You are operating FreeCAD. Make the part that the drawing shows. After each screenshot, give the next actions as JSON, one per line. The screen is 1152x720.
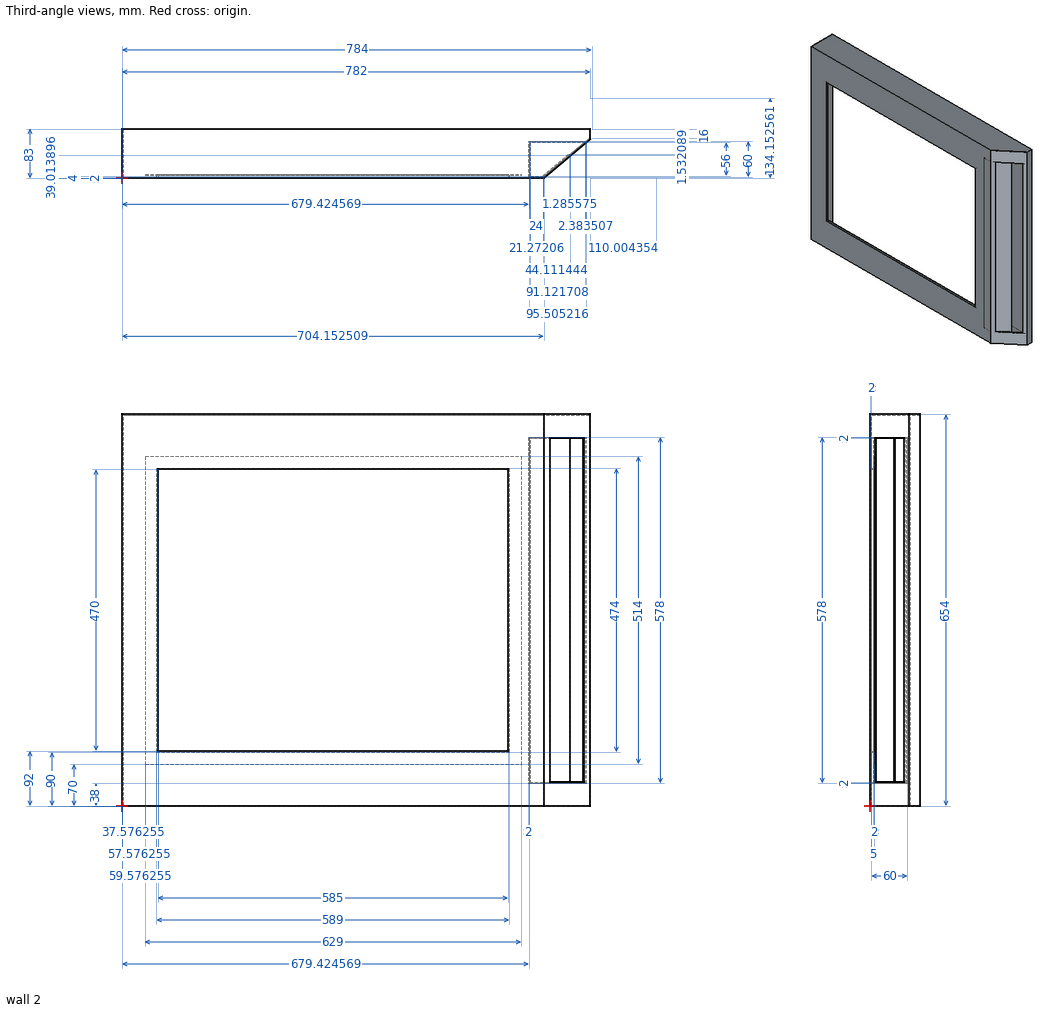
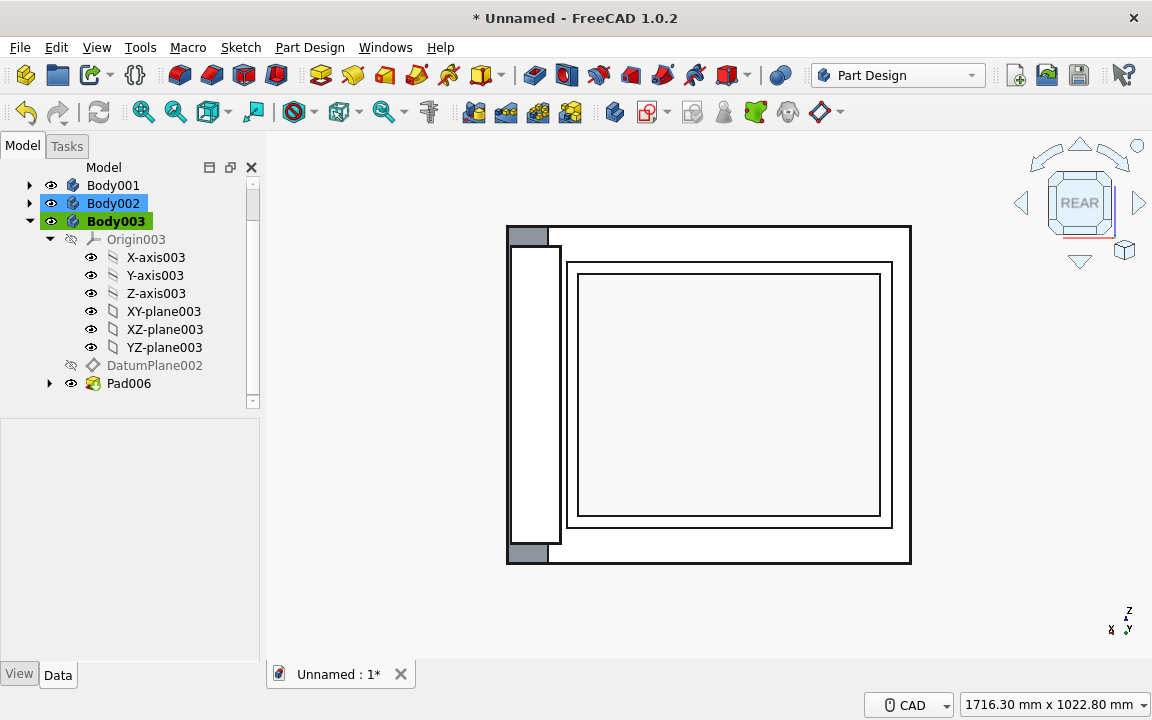
{"action": "key", "text": "0"}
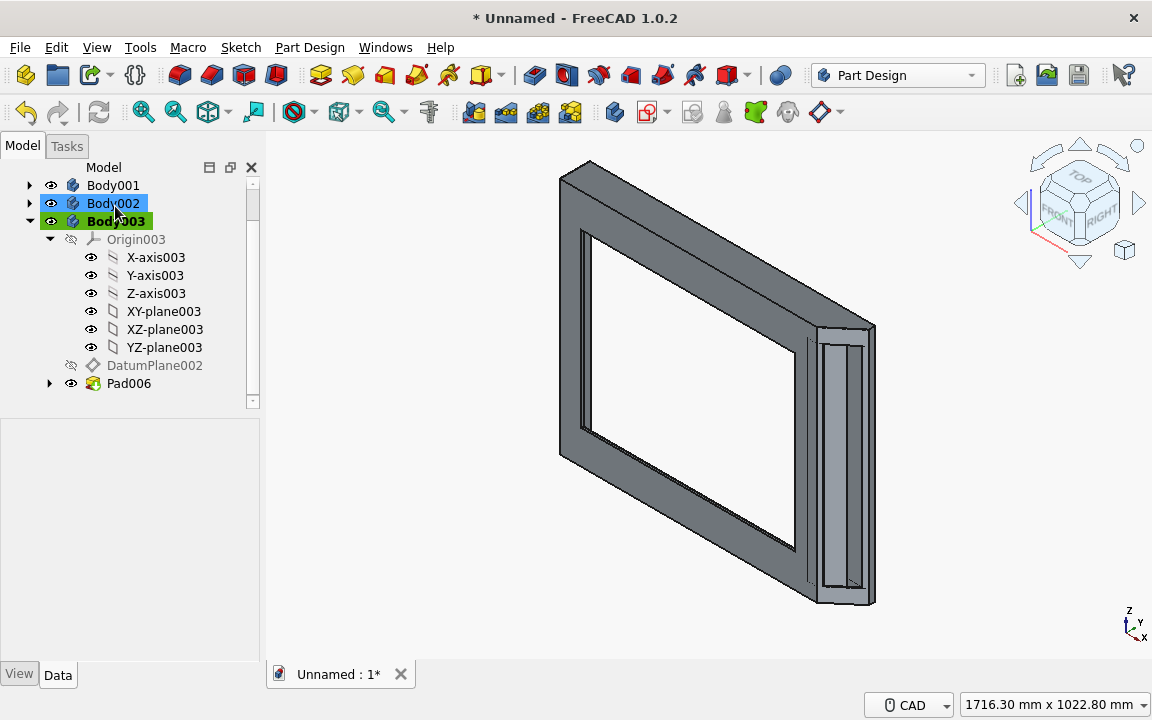
{"action": "key", "text": "v f"}